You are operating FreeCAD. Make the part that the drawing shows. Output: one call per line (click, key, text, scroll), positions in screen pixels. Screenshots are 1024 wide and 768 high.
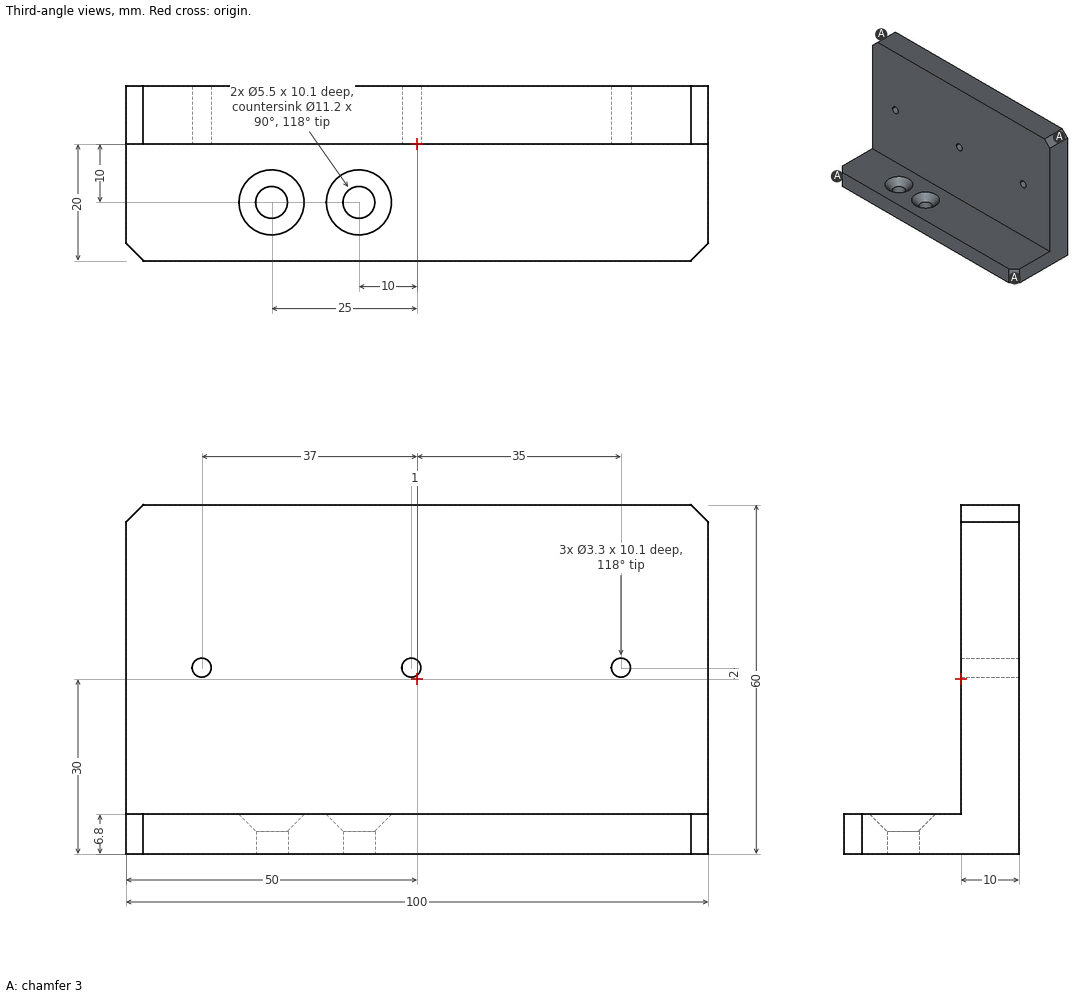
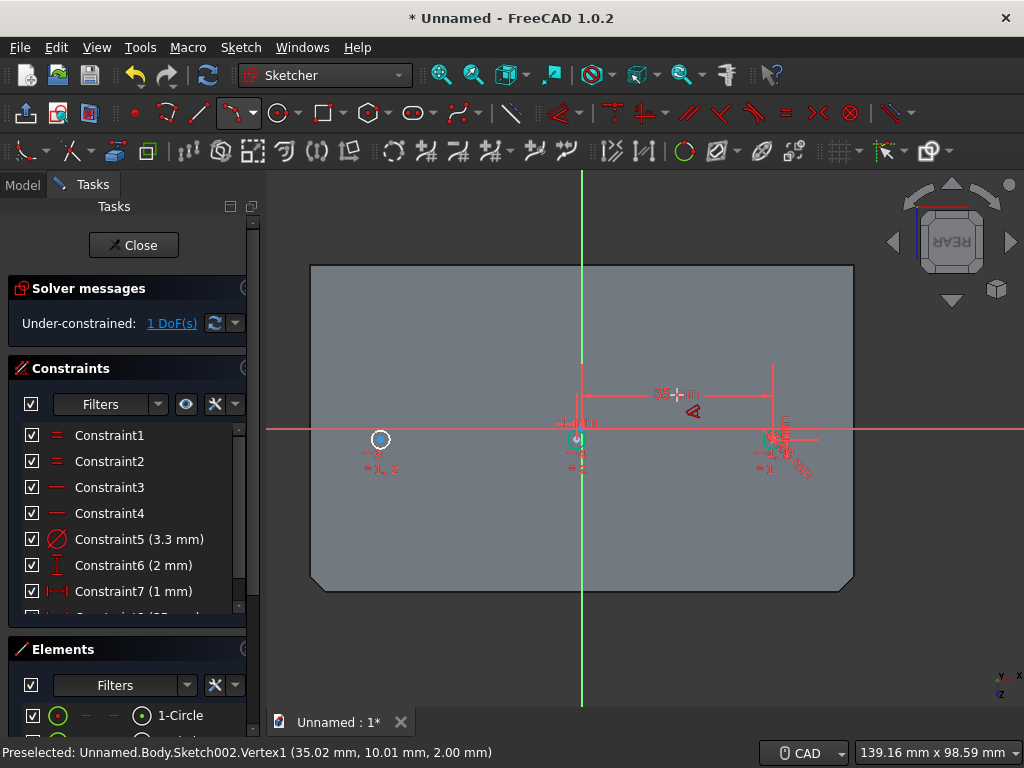
click(381, 440)
click(481, 395)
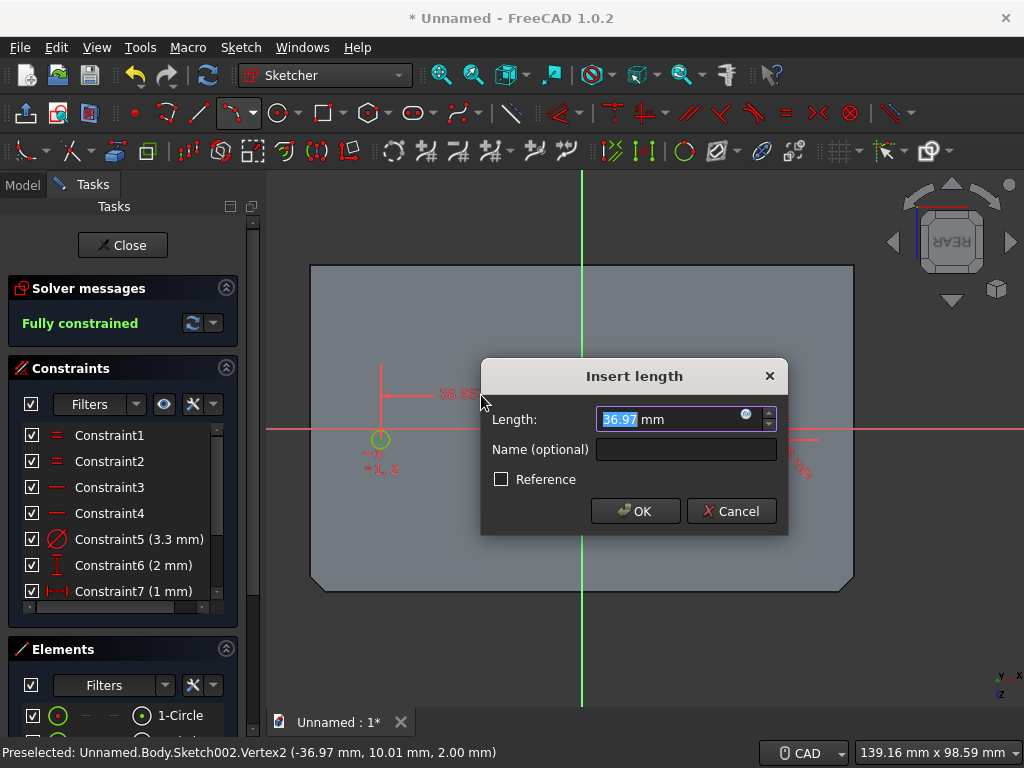
text(37)
key(Return)
key(Escape)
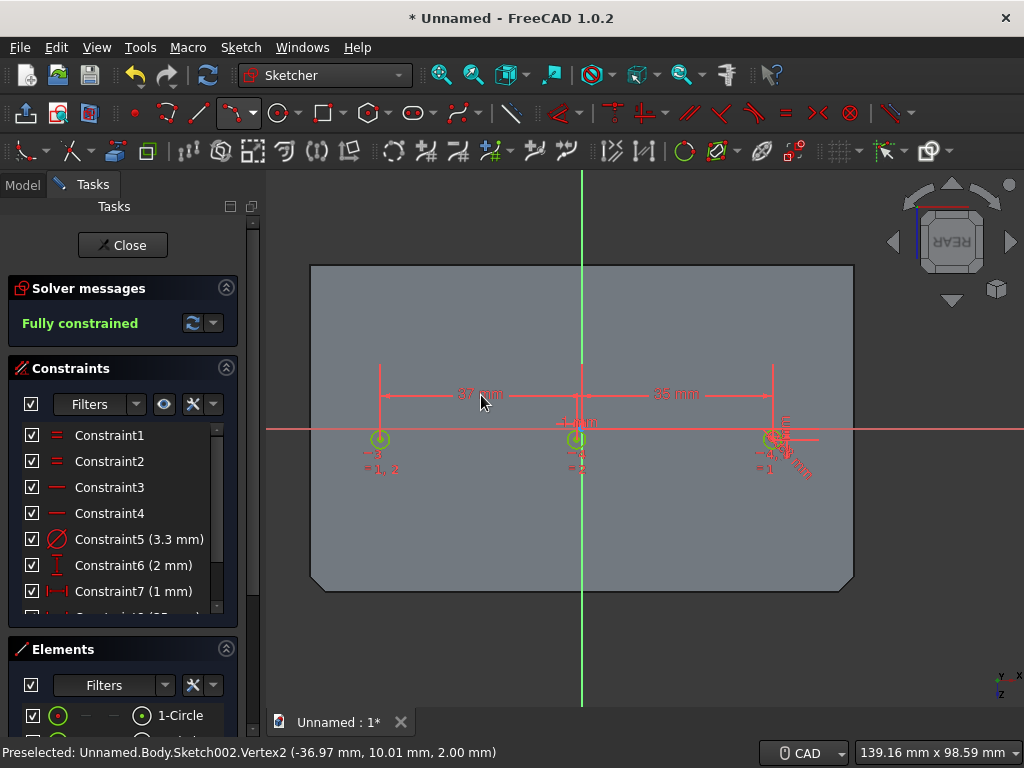
click(123, 245)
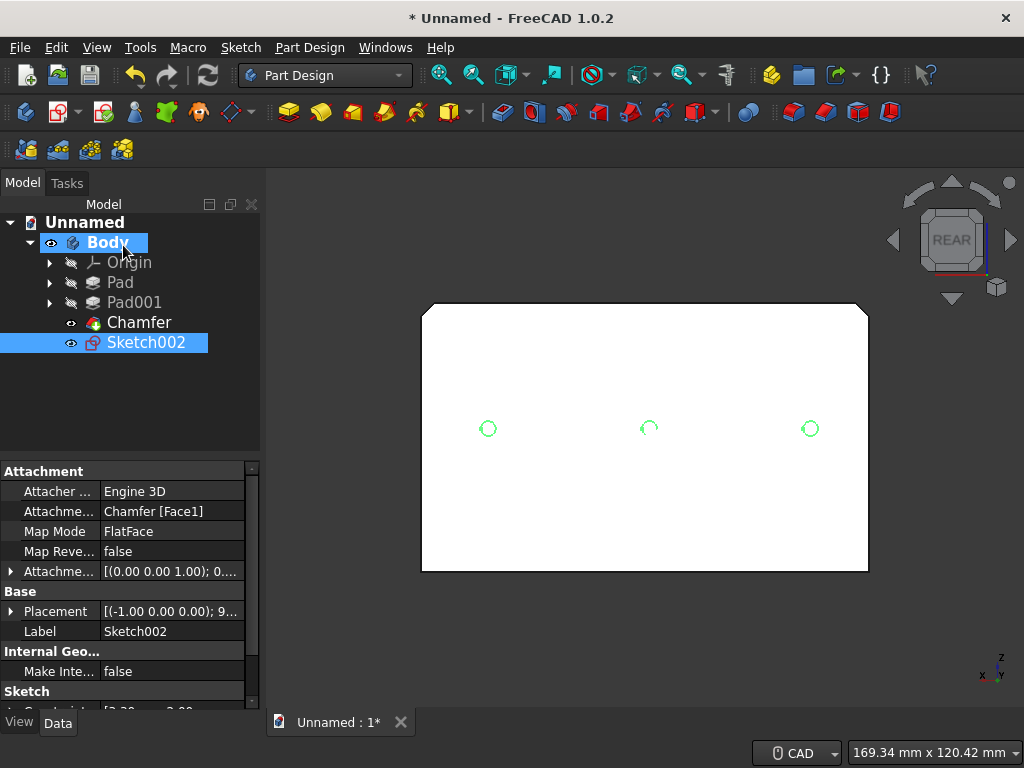
click(536, 112)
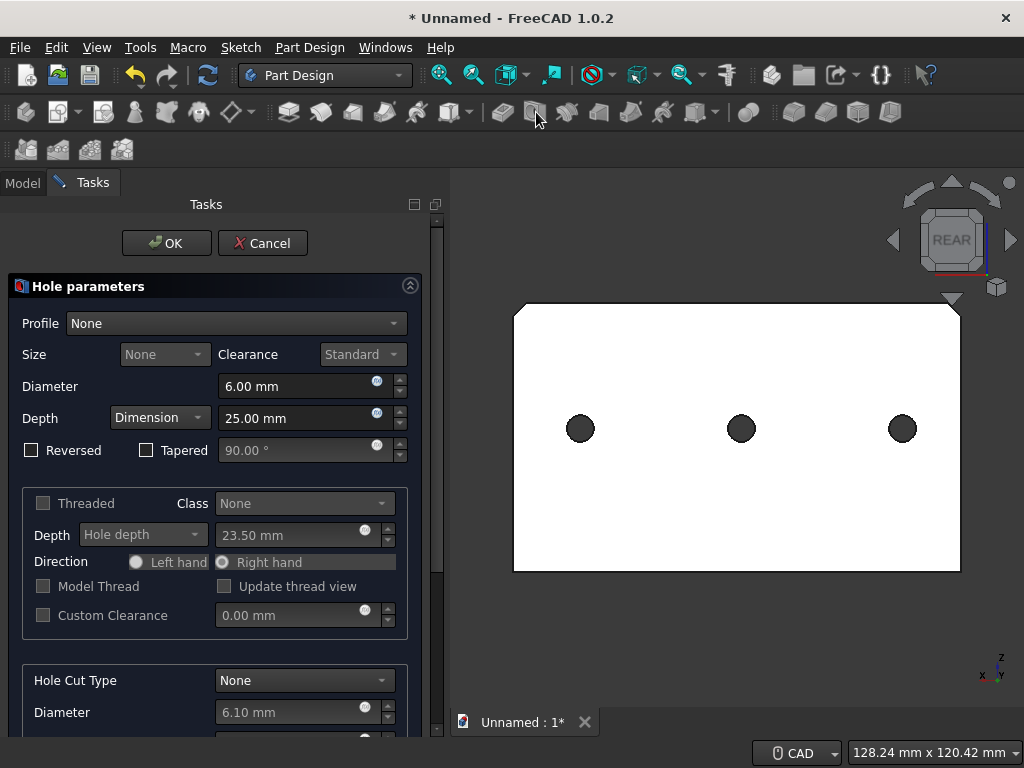
triple_click(305, 386)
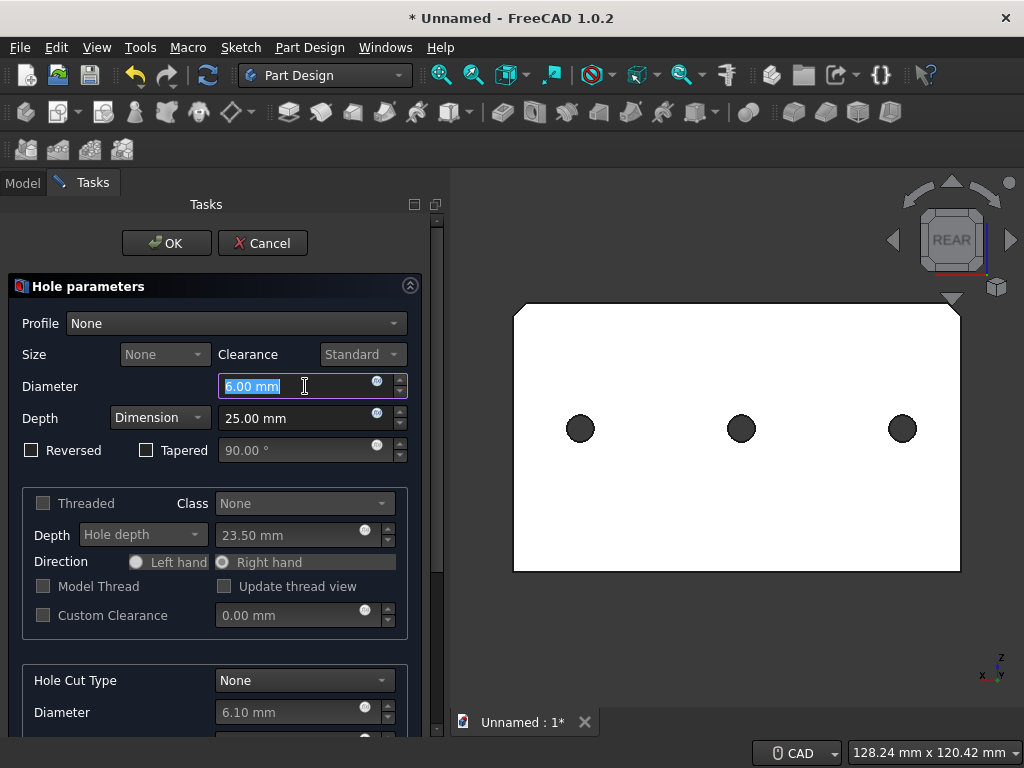
text(3.3)
key(Tab)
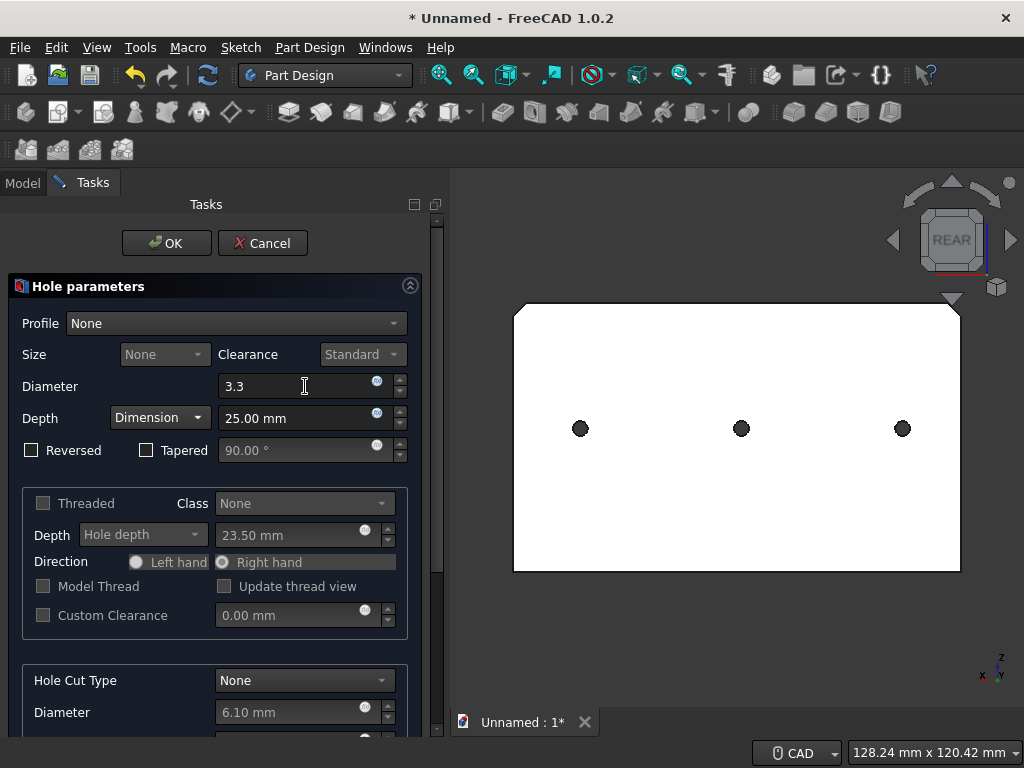
triple_click(305, 418)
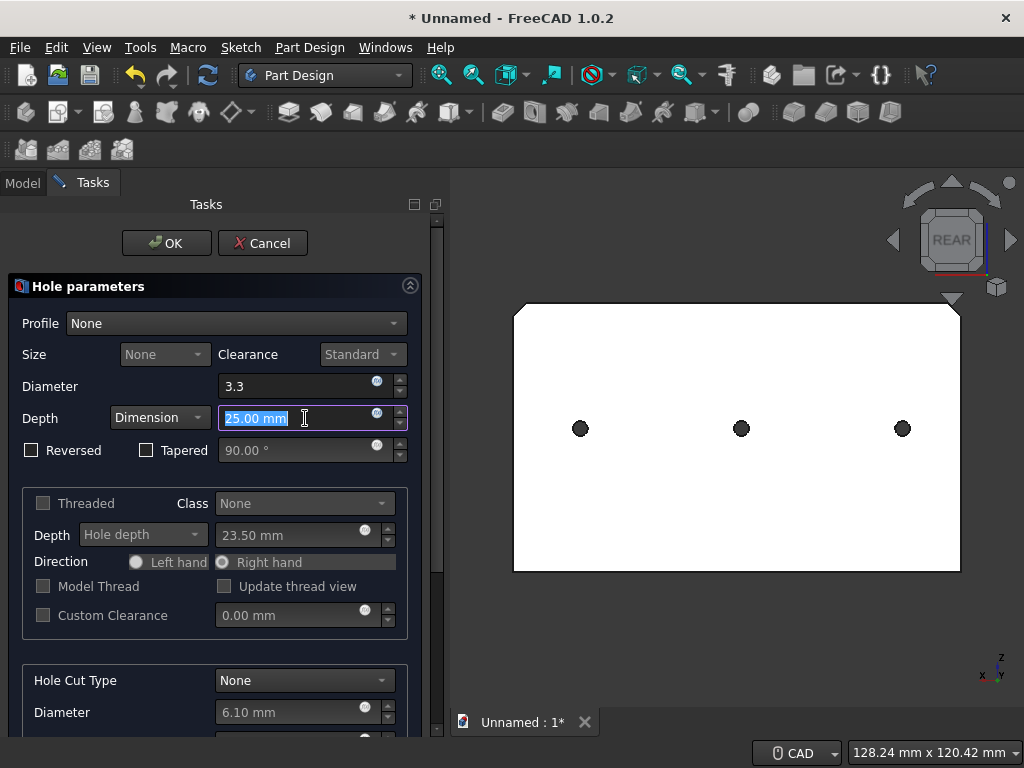
text(10.1)
key(Tab)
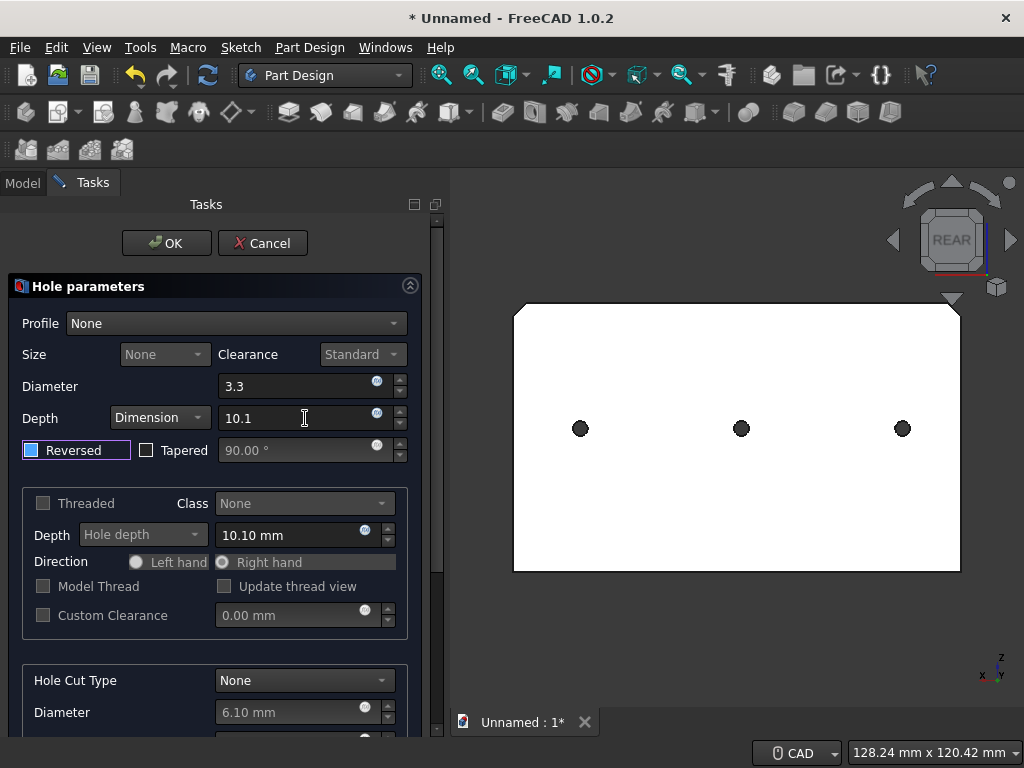
click(167, 243)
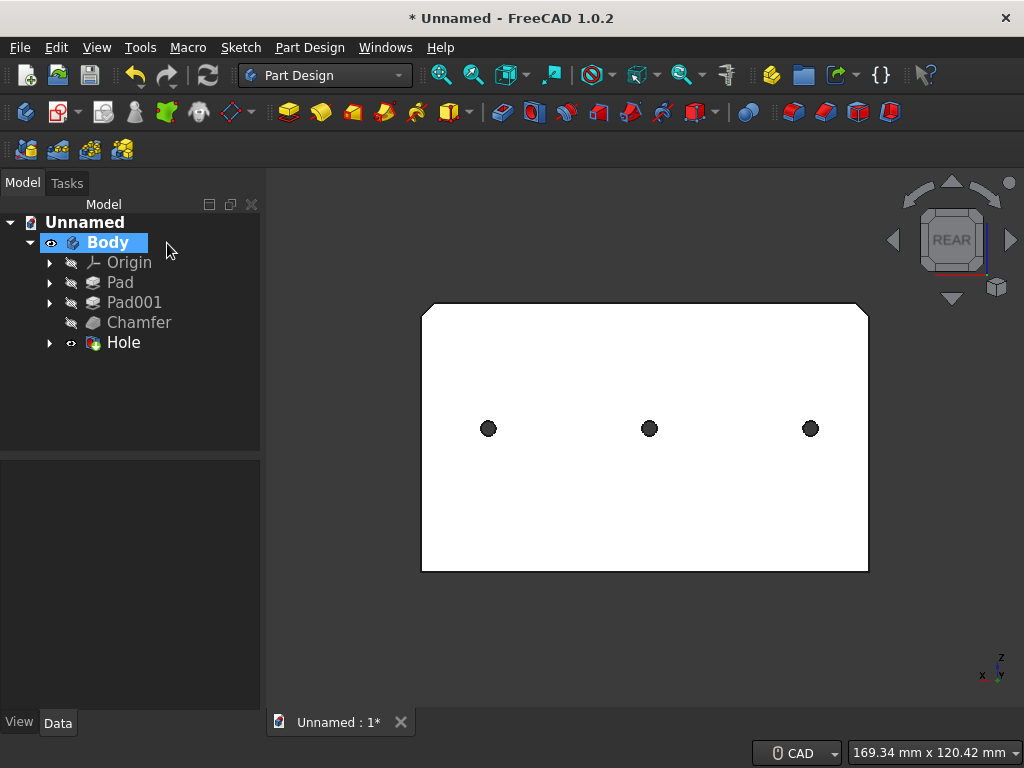
key(0)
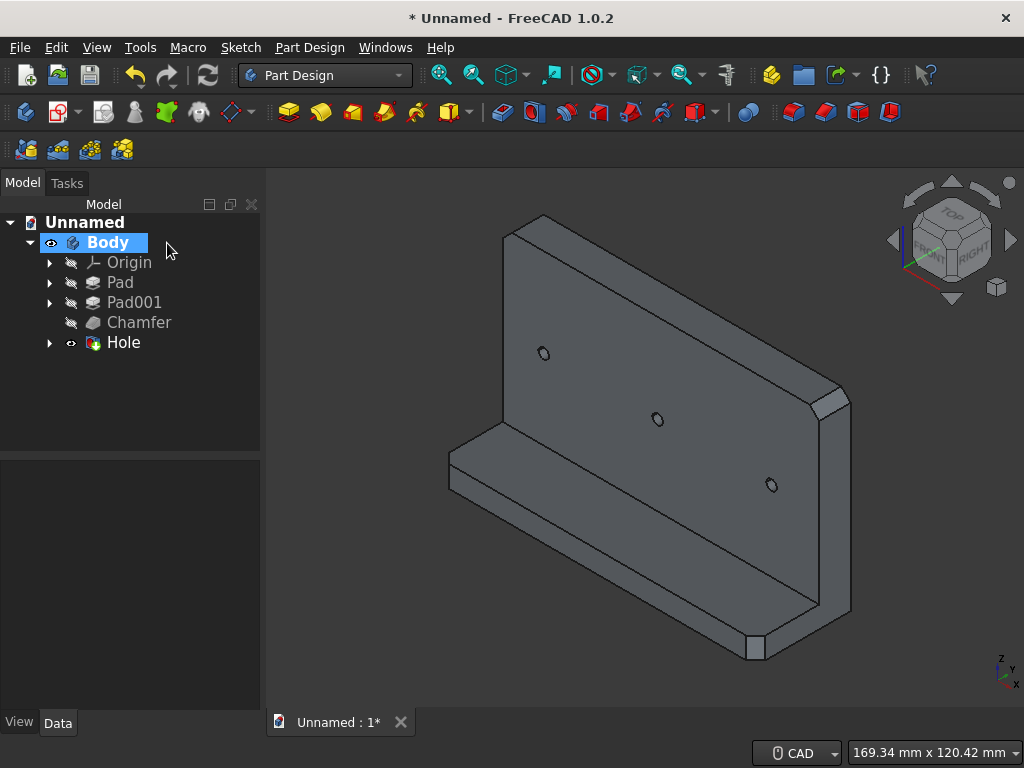
click(720, 583)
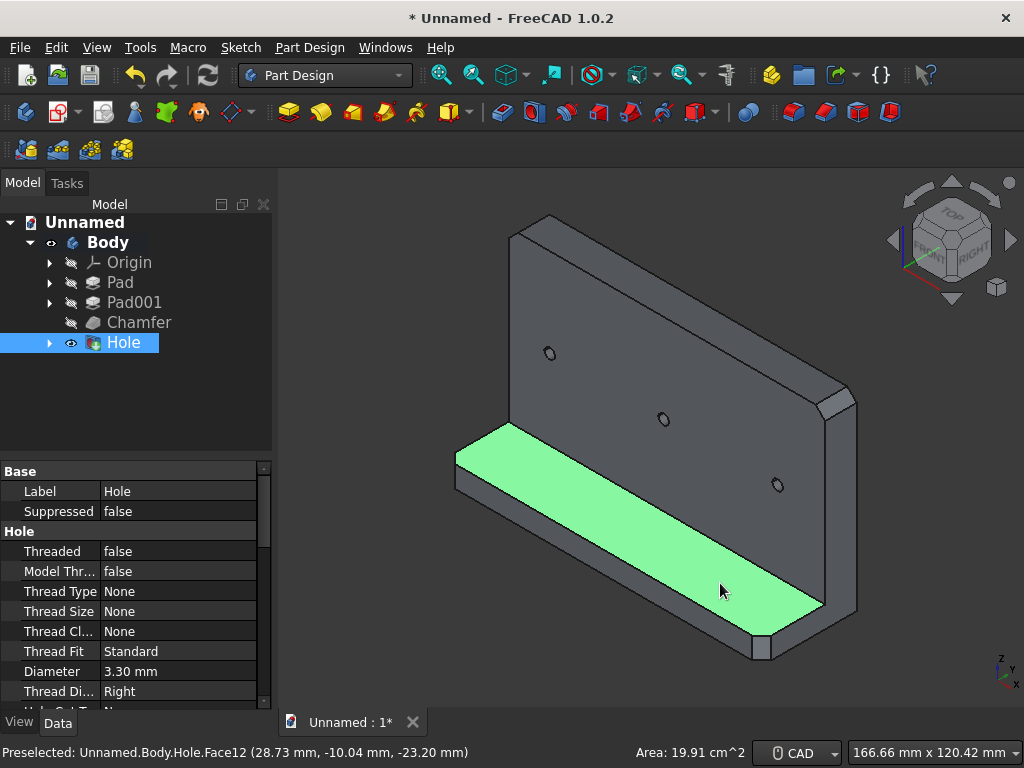
click(58, 112)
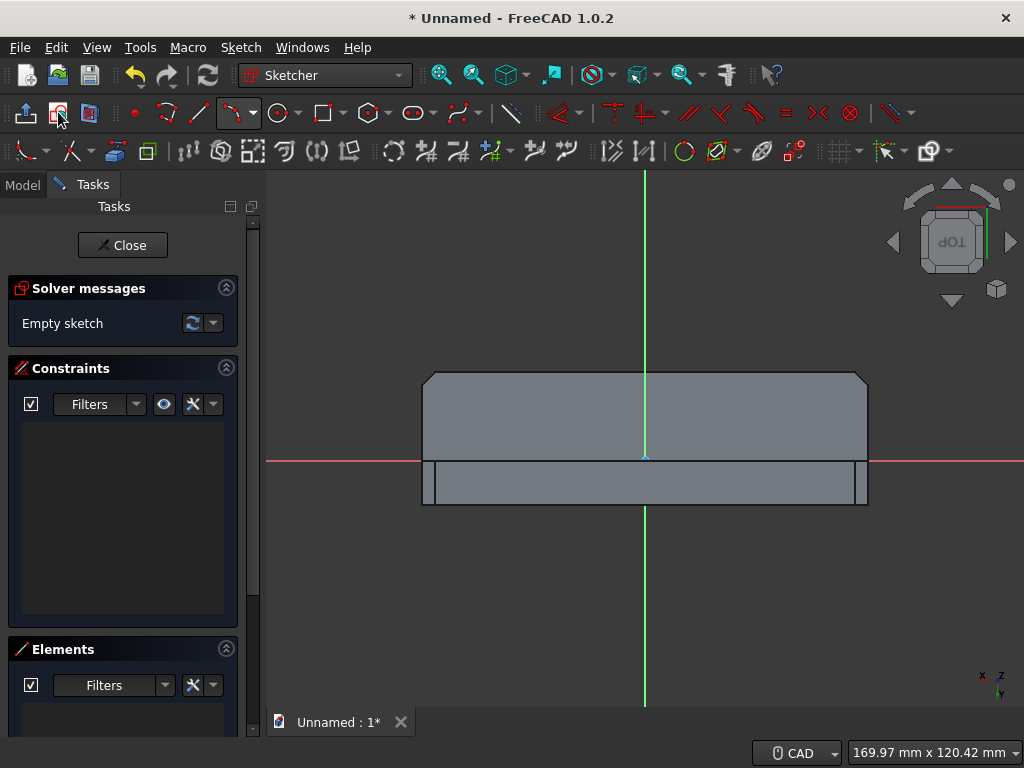
scroll(763, 430, up, 6)